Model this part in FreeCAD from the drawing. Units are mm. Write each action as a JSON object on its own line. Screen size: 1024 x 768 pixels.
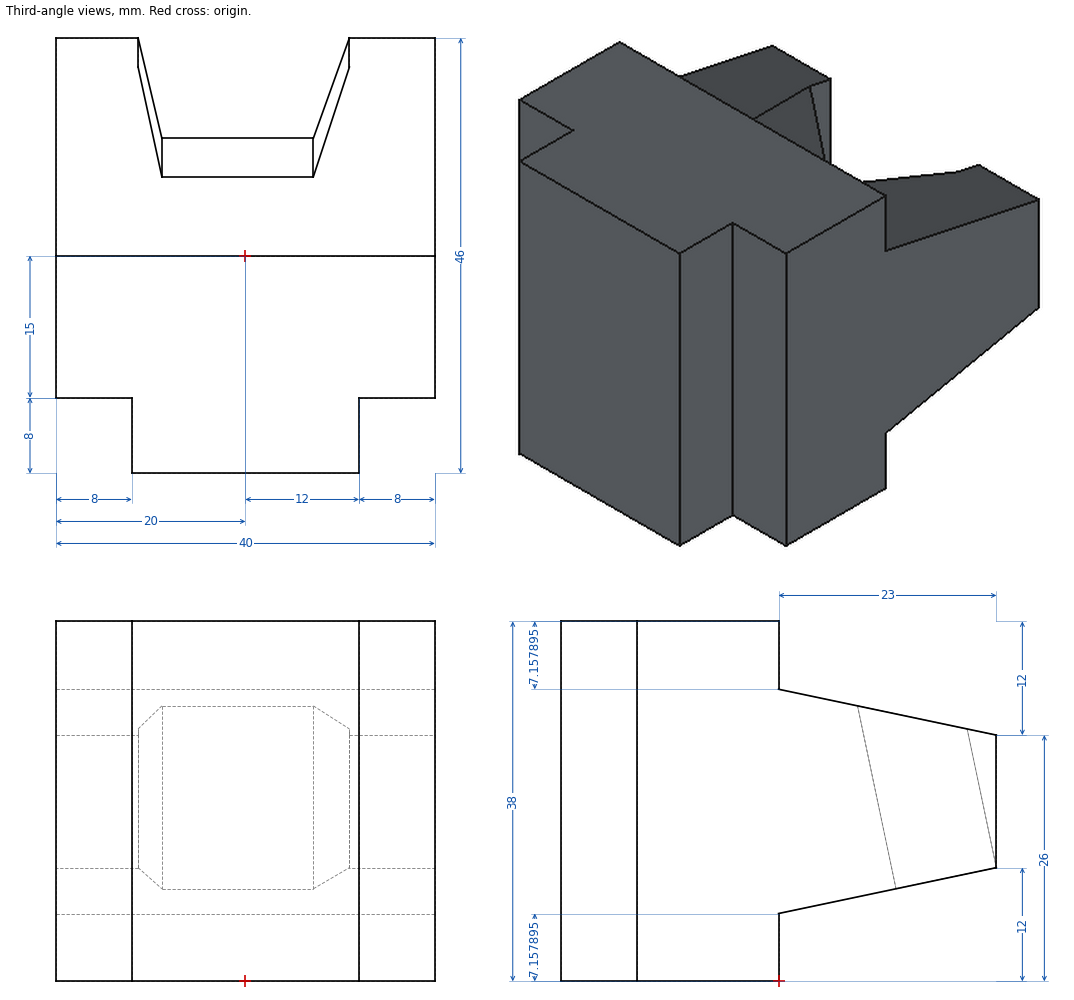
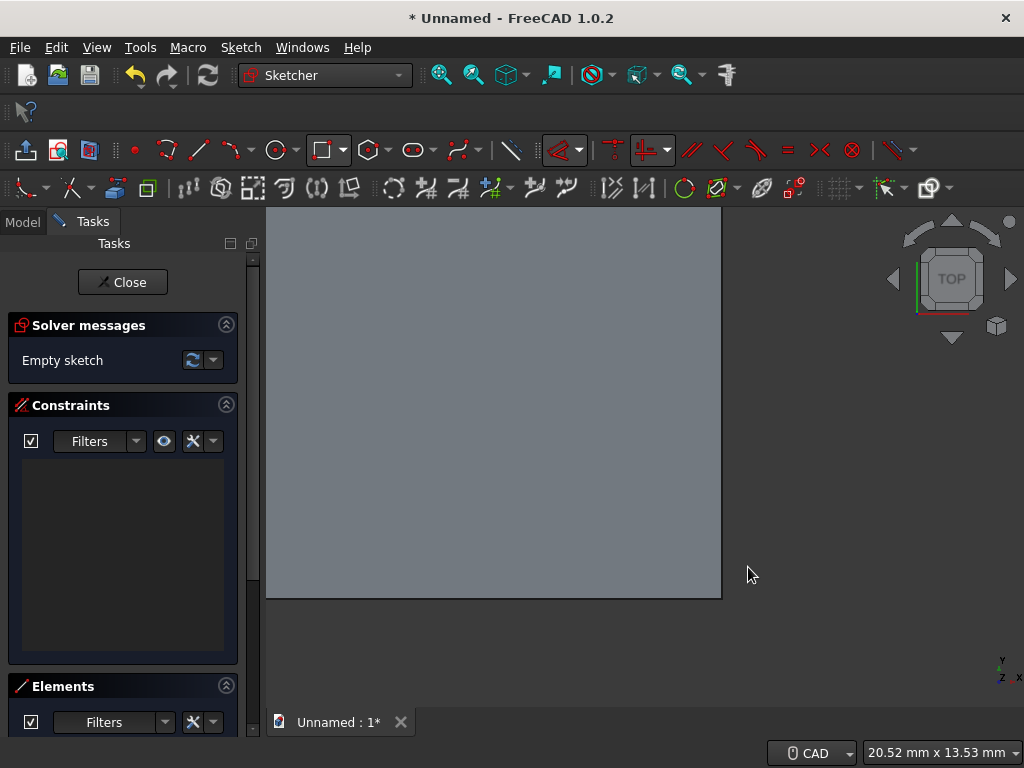
{"action": "left_click", "coordinate": [322, 150]}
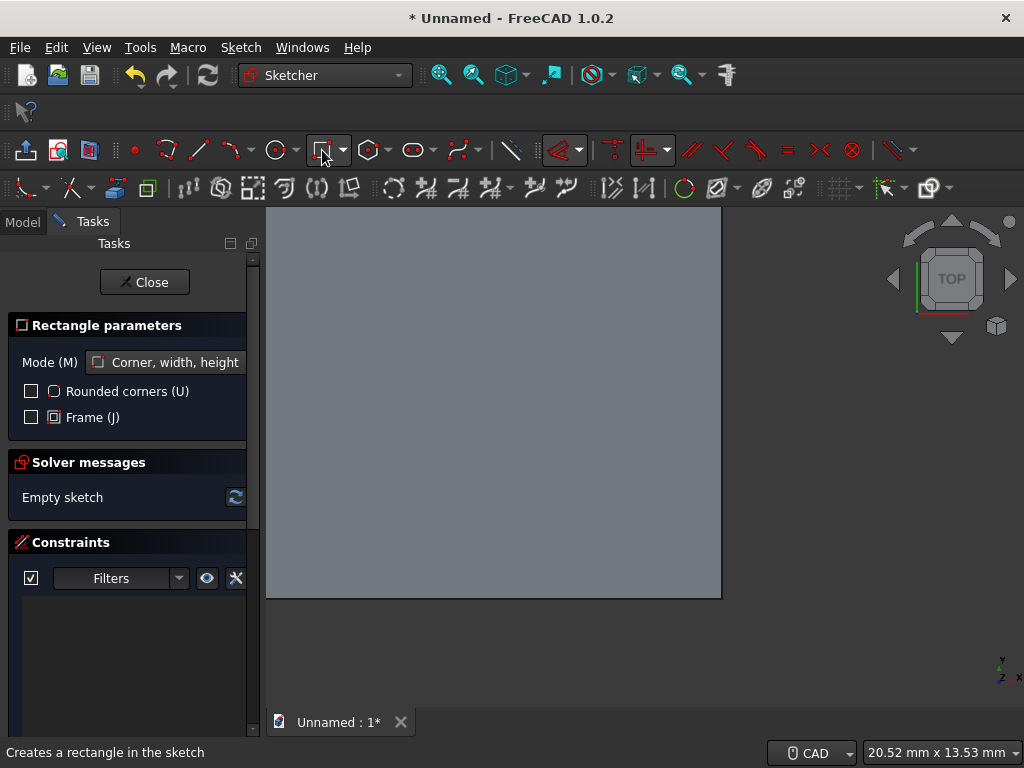
{"action": "left_click", "coordinate": [426, 304]}
{"action": "left_click", "coordinate": [722, 599]}
{"action": "key", "text": "Escape"}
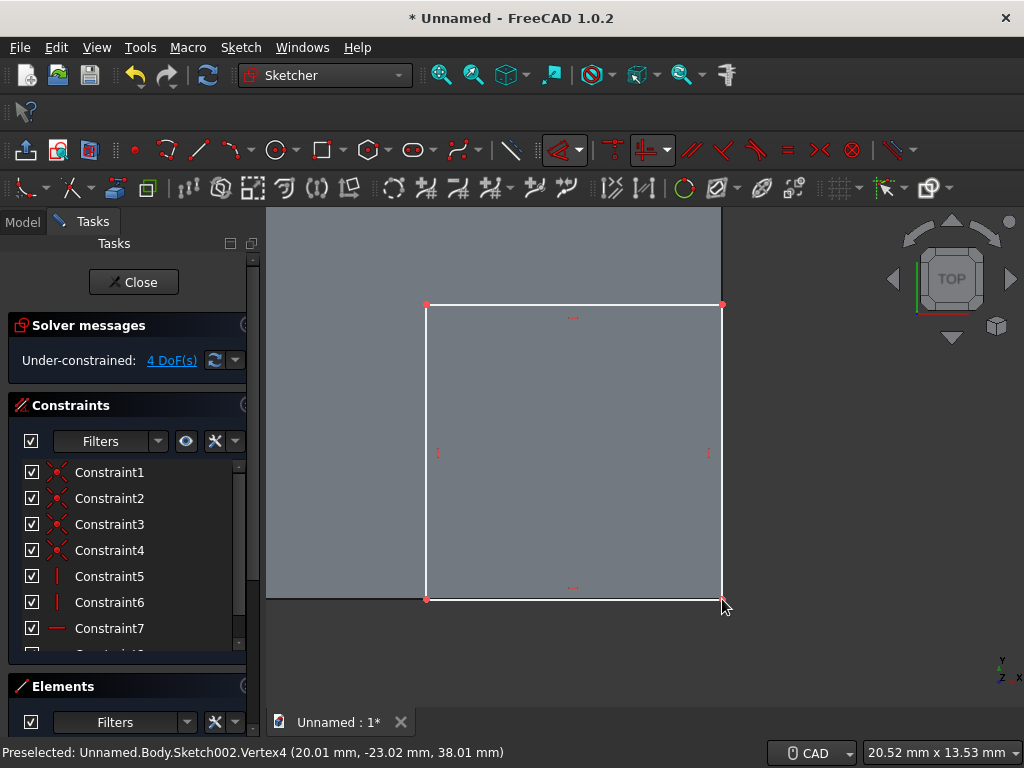
{"action": "left_click", "coordinate": [426, 393]}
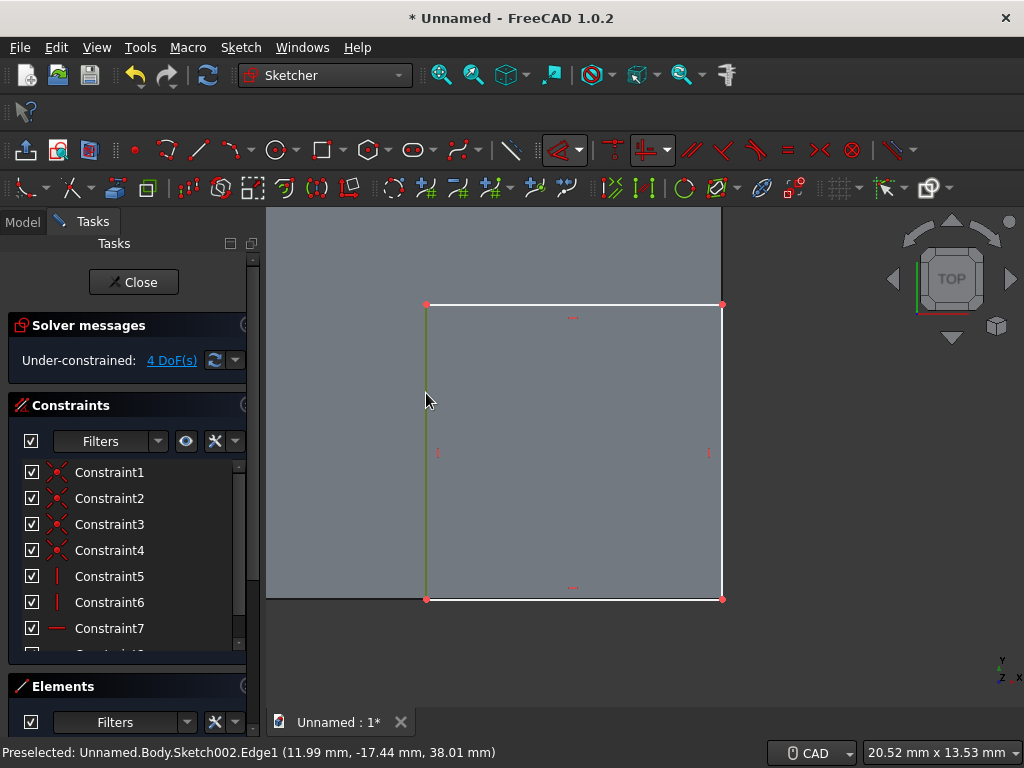
{"action": "left_click", "coordinate": [582, 150]}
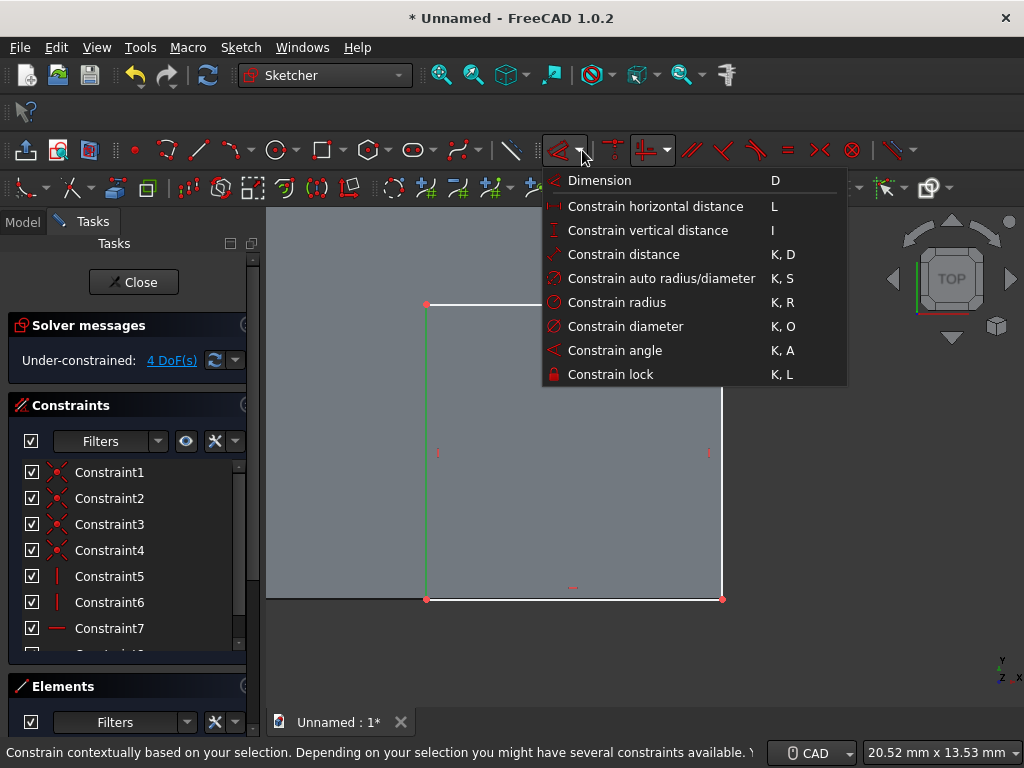
{"action": "left_click", "coordinate": [695, 230]}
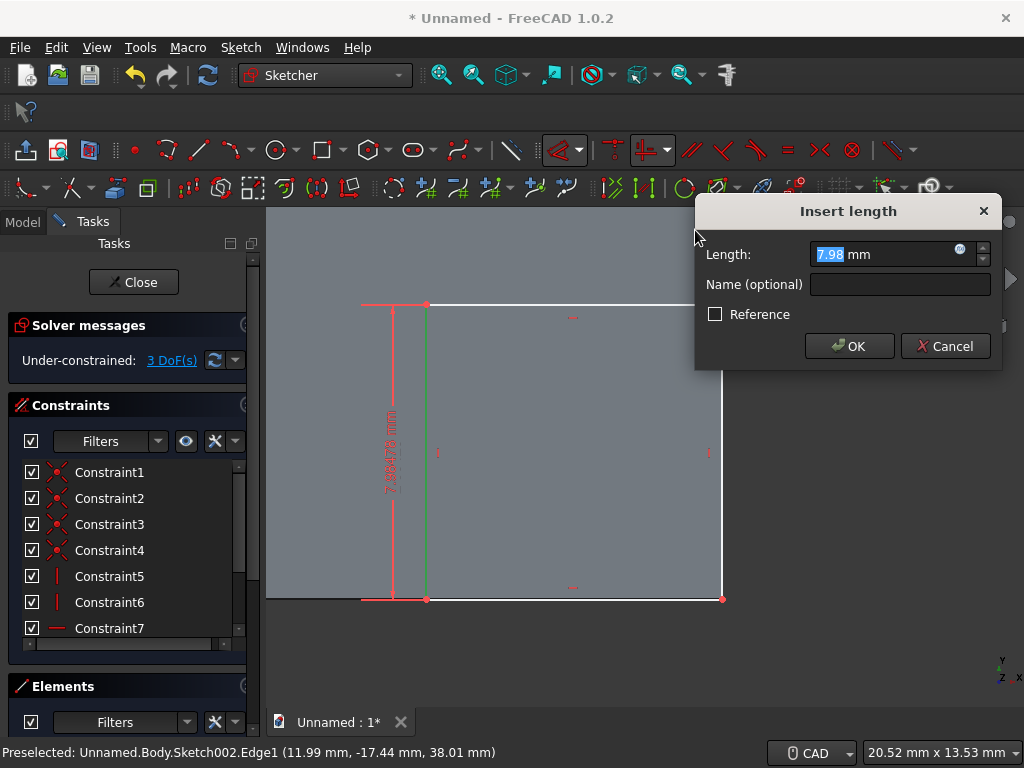
{"action": "type", "text": "8"}
{"action": "key", "text": "Return"}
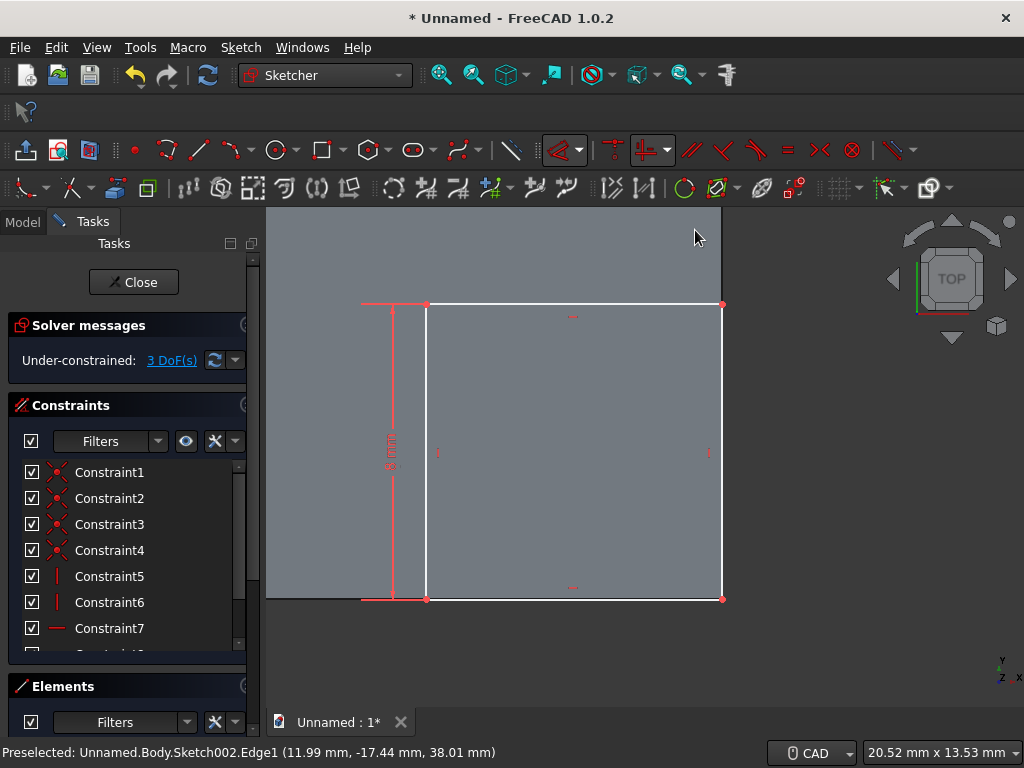
{"action": "left_click", "coordinate": [515, 600]}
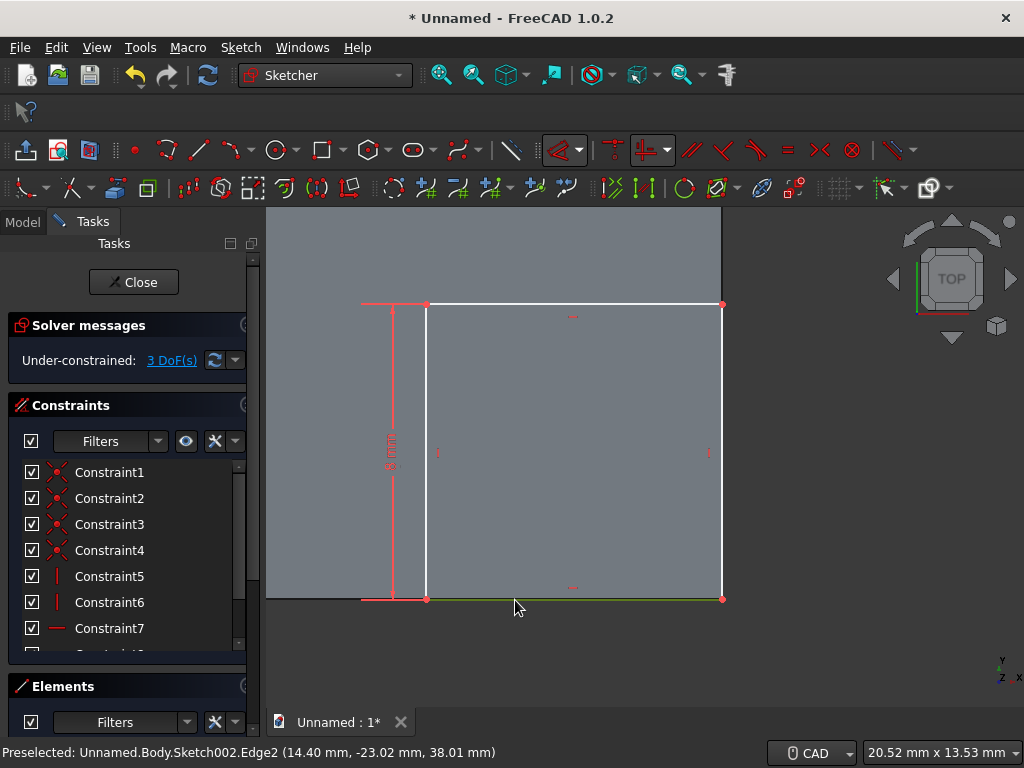
{"action": "left_click", "coordinate": [582, 150]}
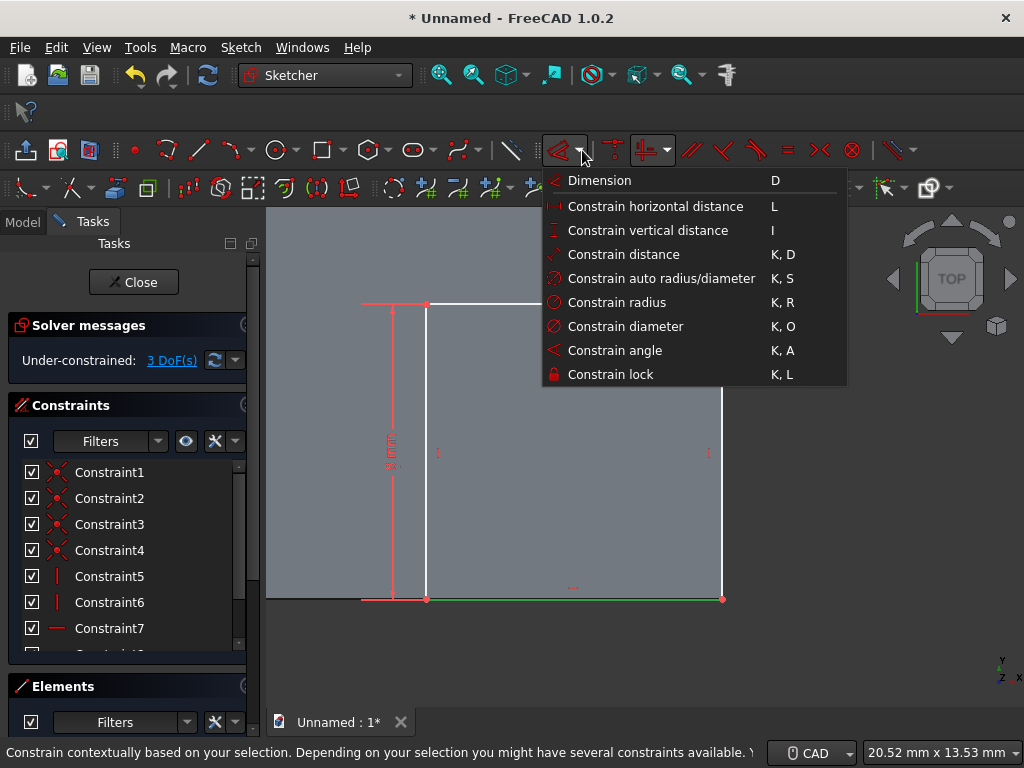
{"action": "left_click", "coordinate": [695, 206]}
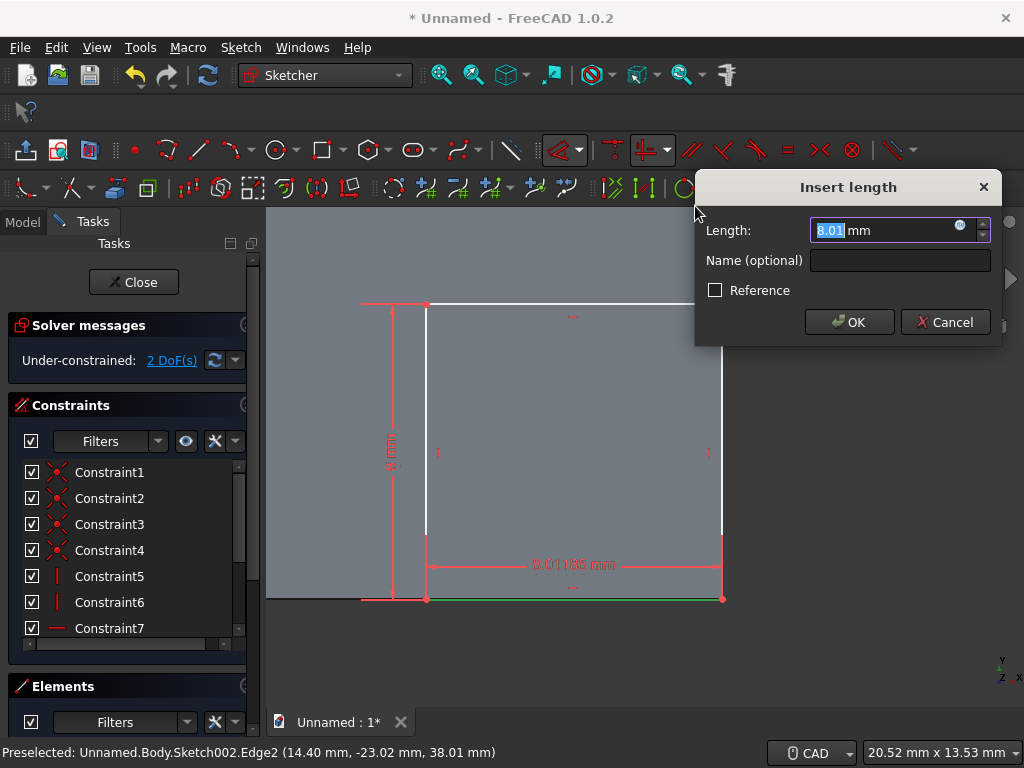
{"action": "type", "text": "8"}
{"action": "key", "text": "Return"}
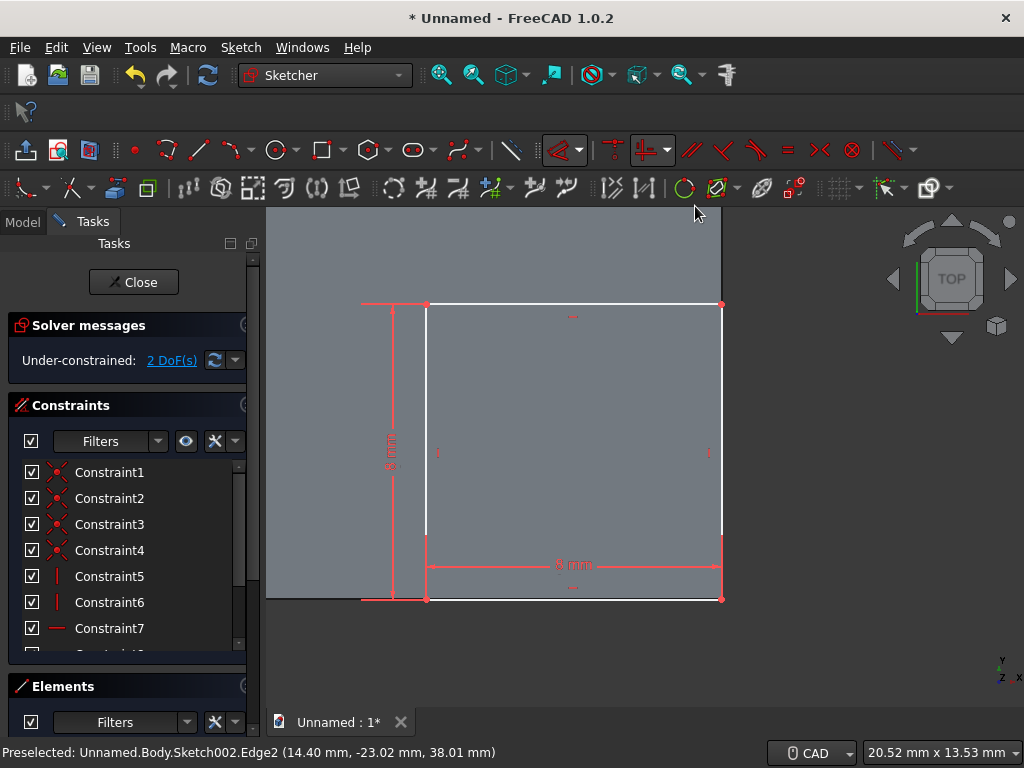
{"action": "left_click", "coordinate": [426, 304]}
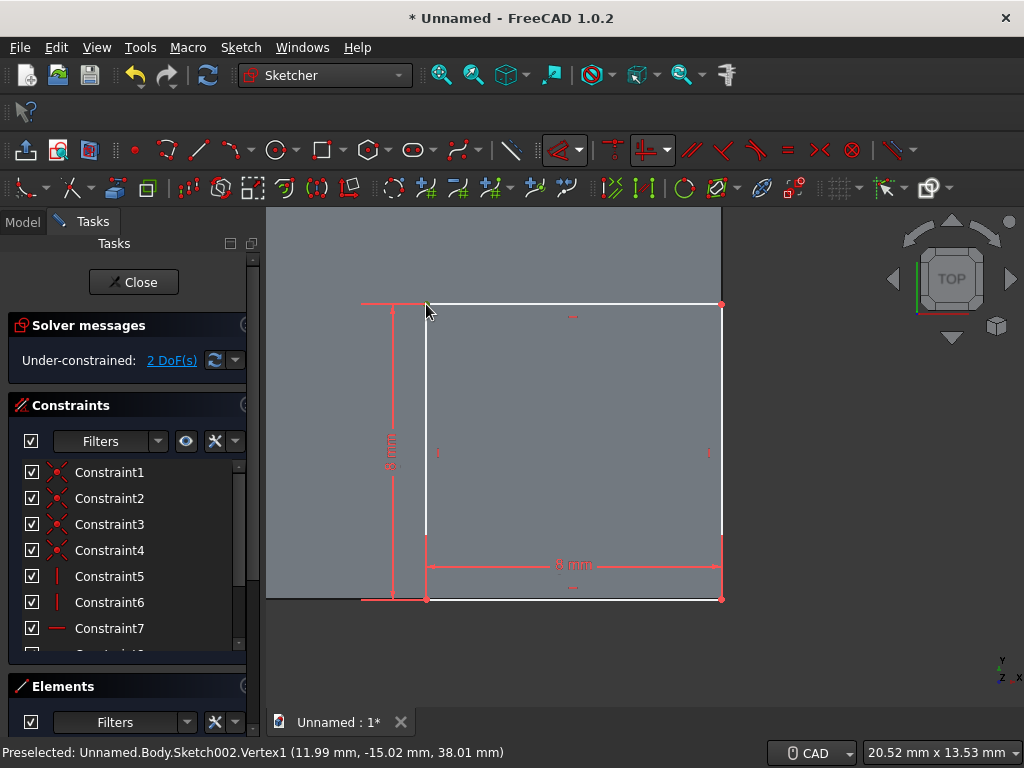
{"action": "left_click", "coordinate": [582, 150]}